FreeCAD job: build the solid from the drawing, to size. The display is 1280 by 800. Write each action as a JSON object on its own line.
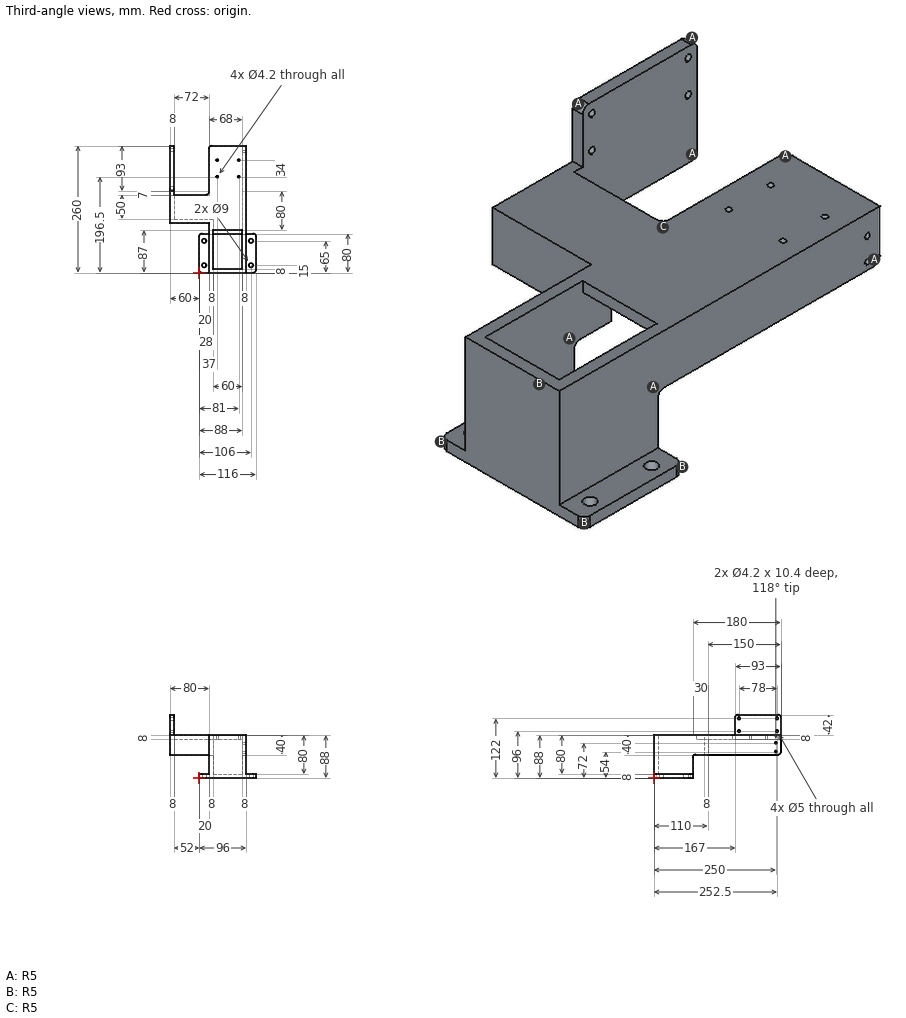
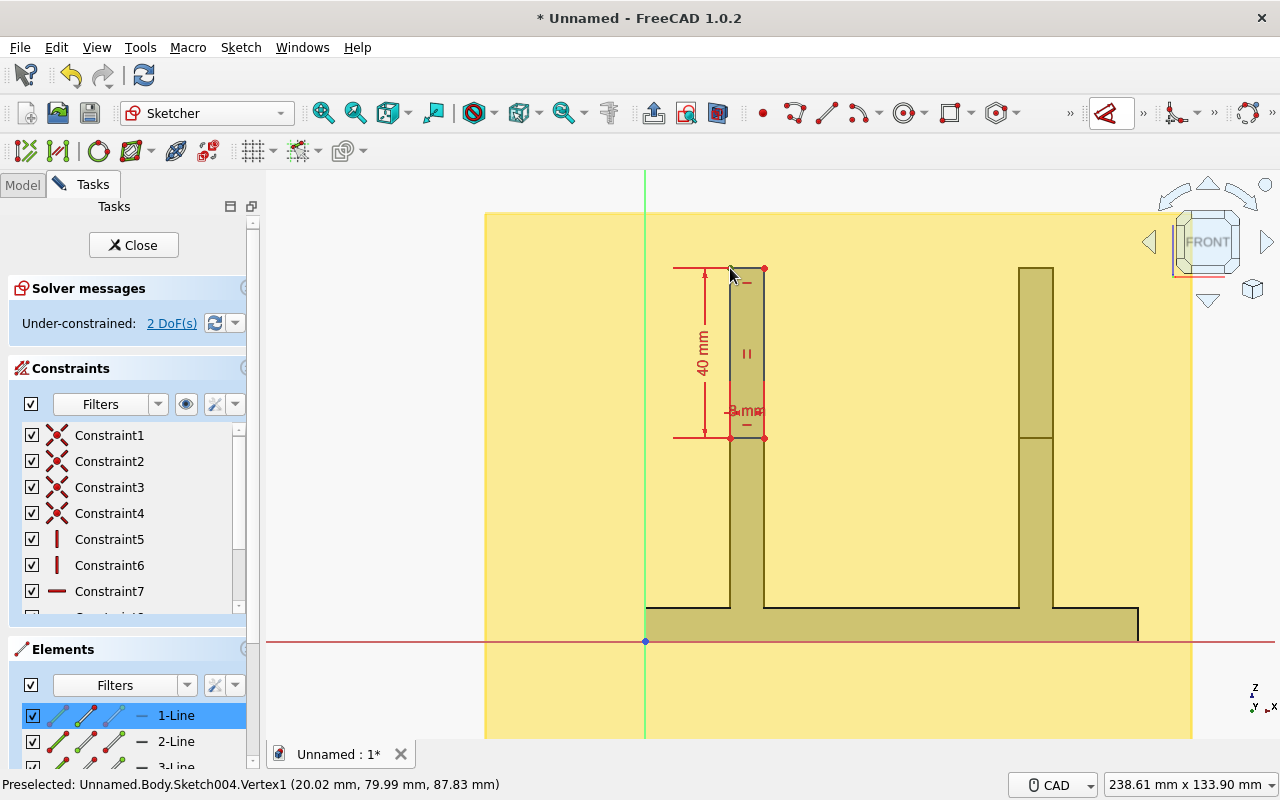
{"action": "left_click", "coordinate": [1128, 114]}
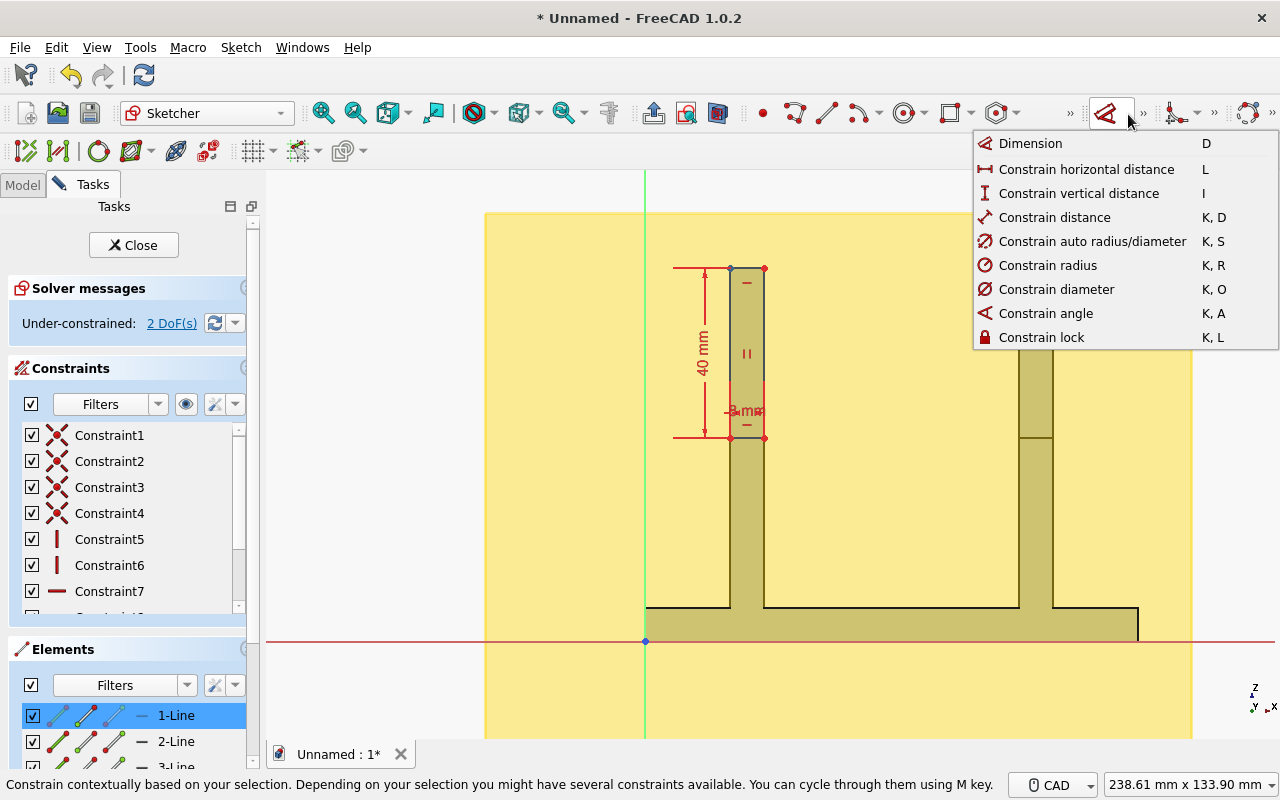
{"action": "left_click", "coordinate": [1126, 169]}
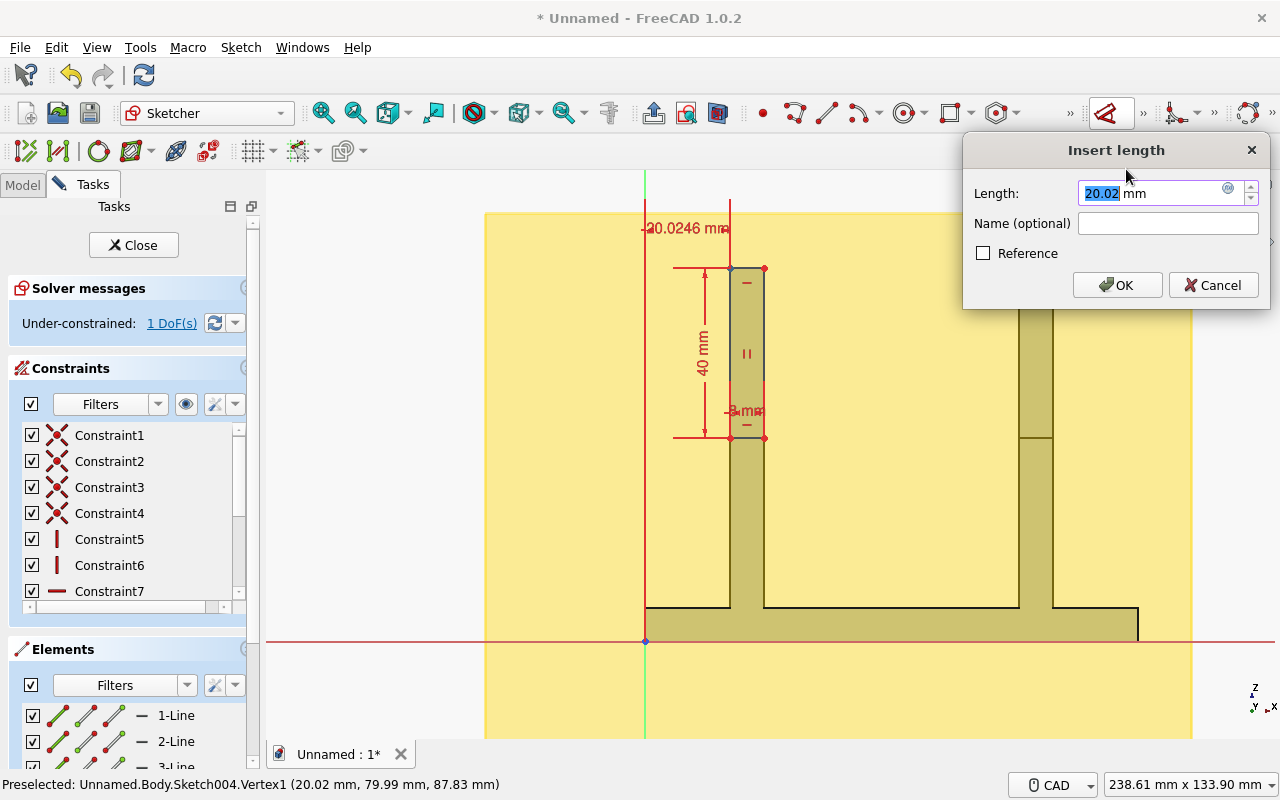
{"action": "type", "text": "20"}
{"action": "key", "text": "Return"}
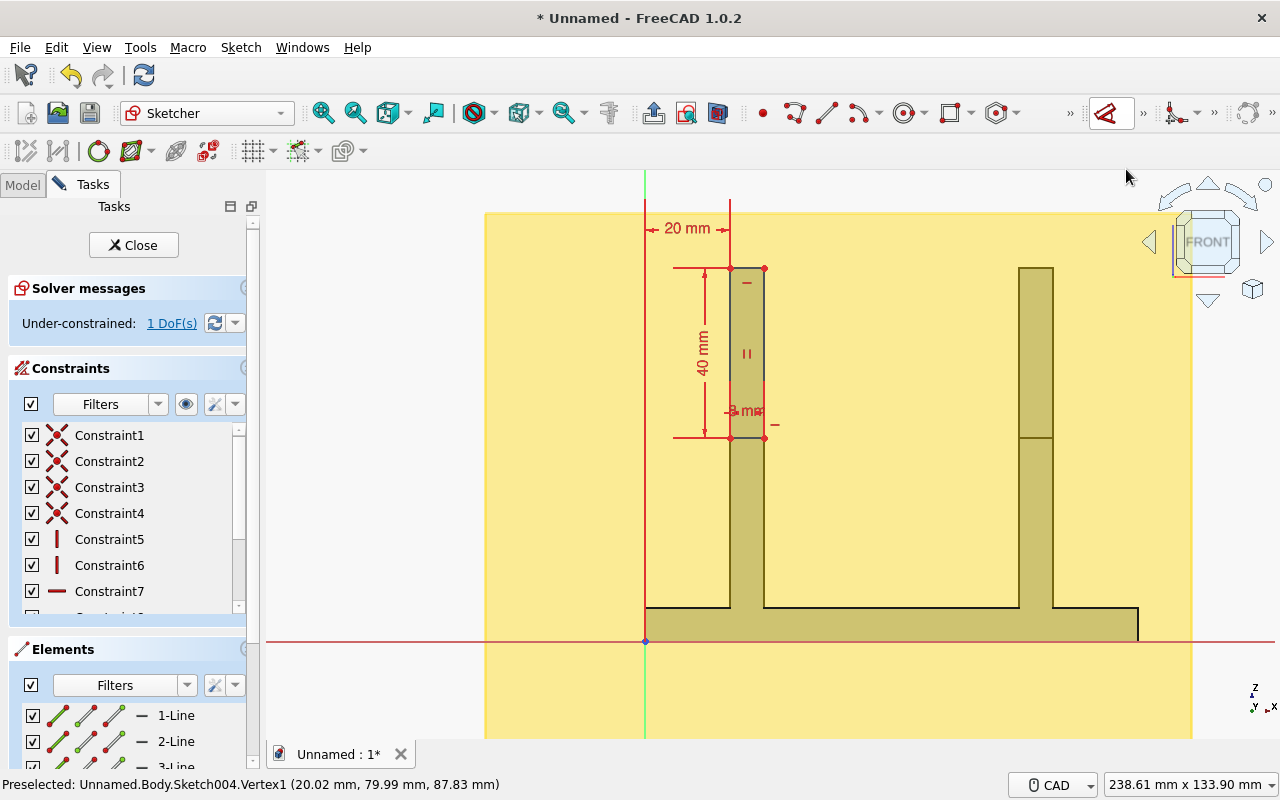
{"action": "left_click", "coordinate": [730, 268]}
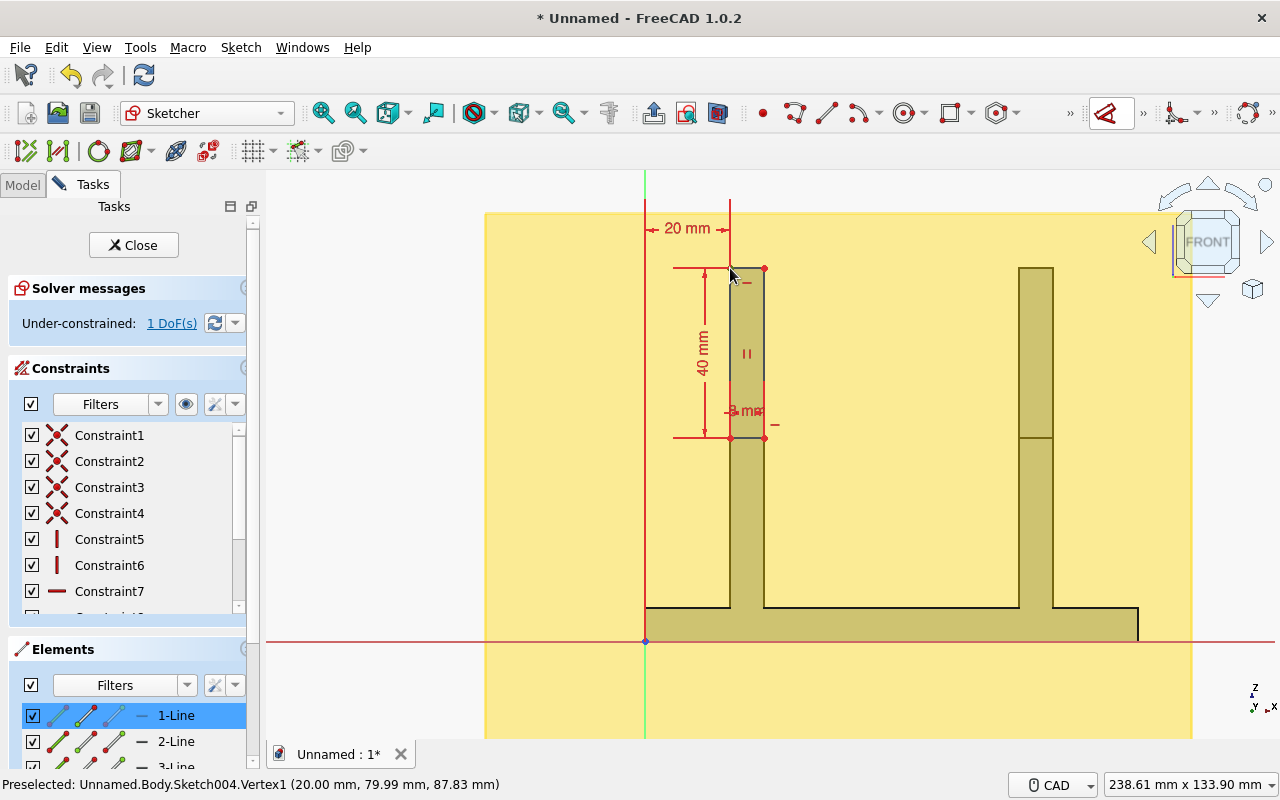
{"action": "key", "text": "i"}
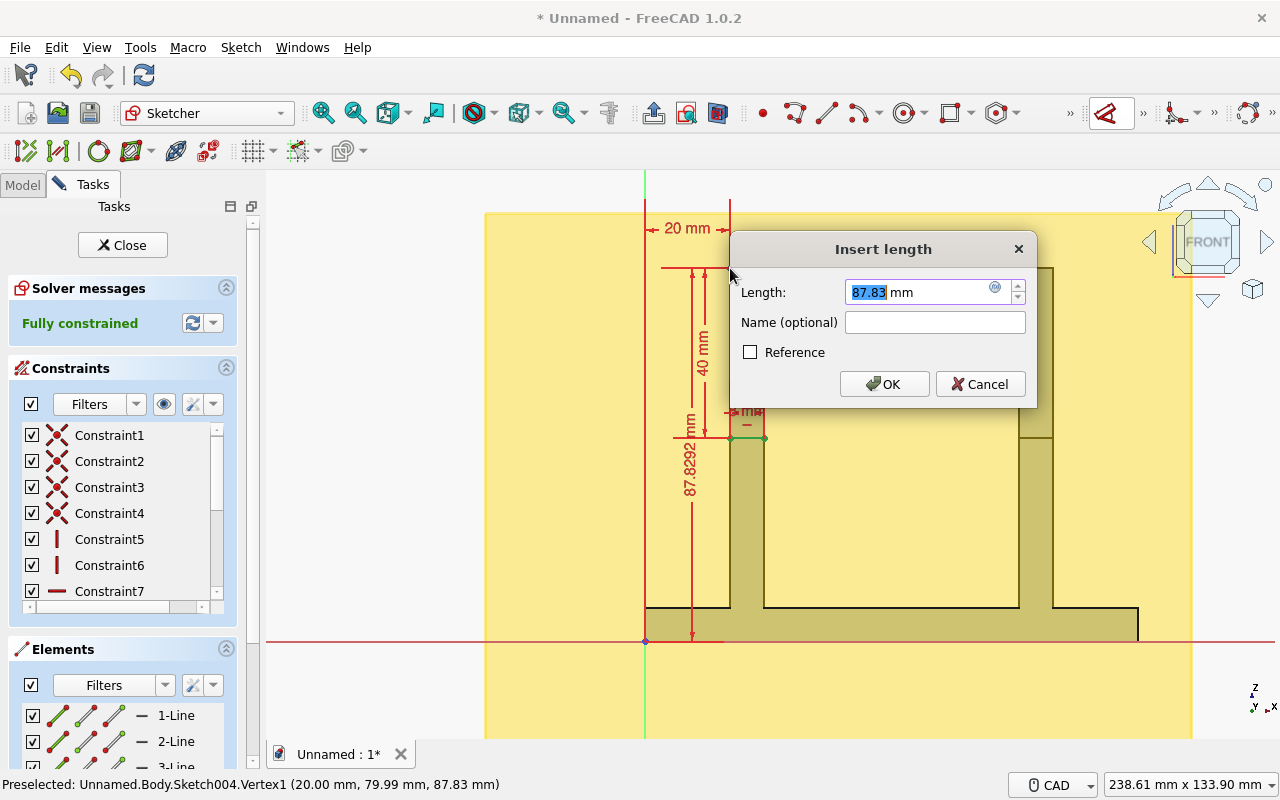
{"action": "type", "text": "88"}
{"action": "key", "text": "Return"}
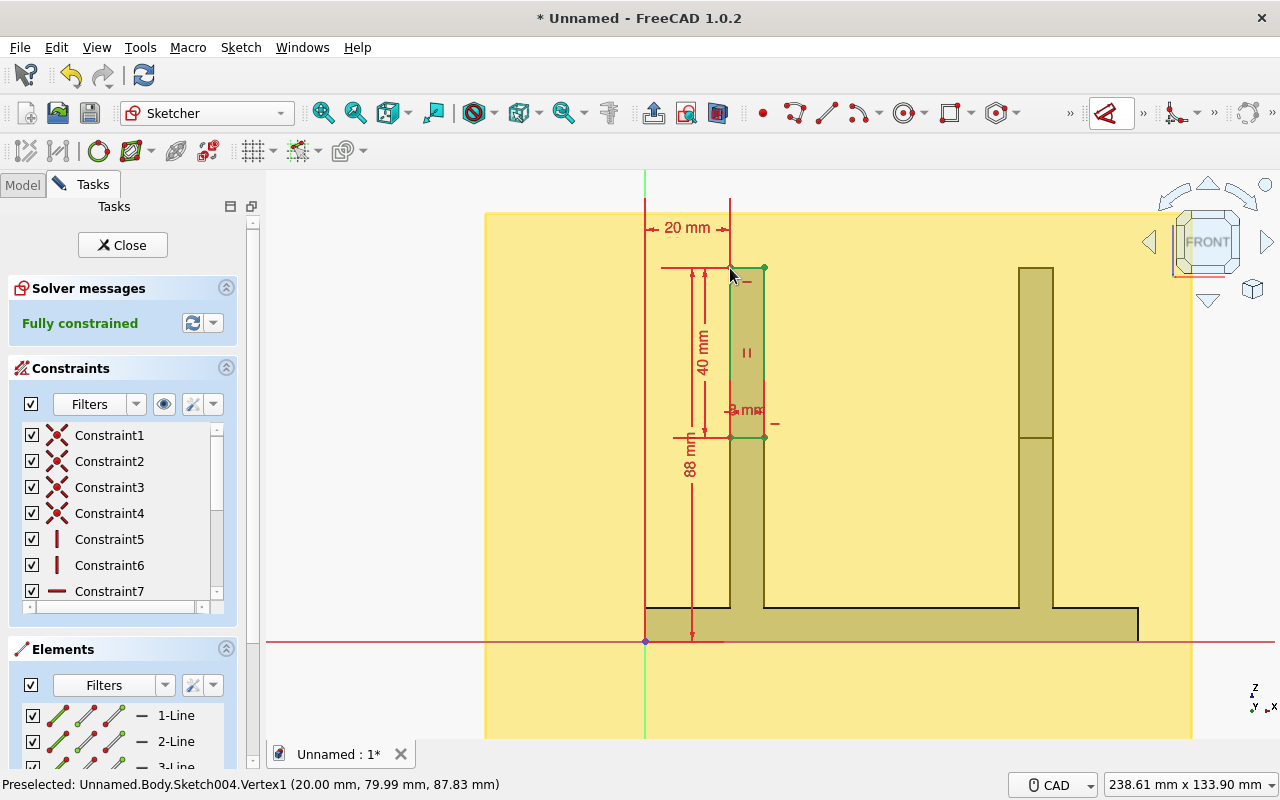
{"action": "left_click", "coordinate": [123, 245]}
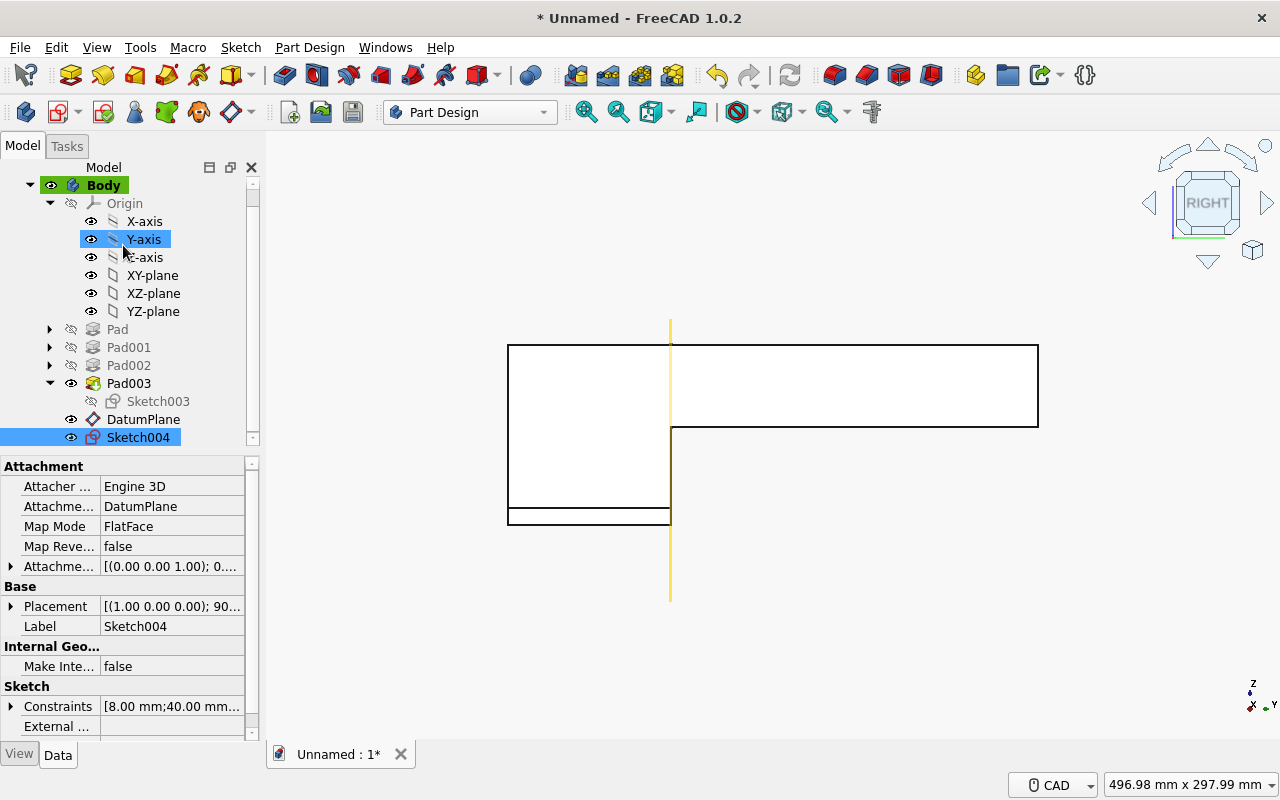
{"action": "left_click", "coordinate": [72, 76]}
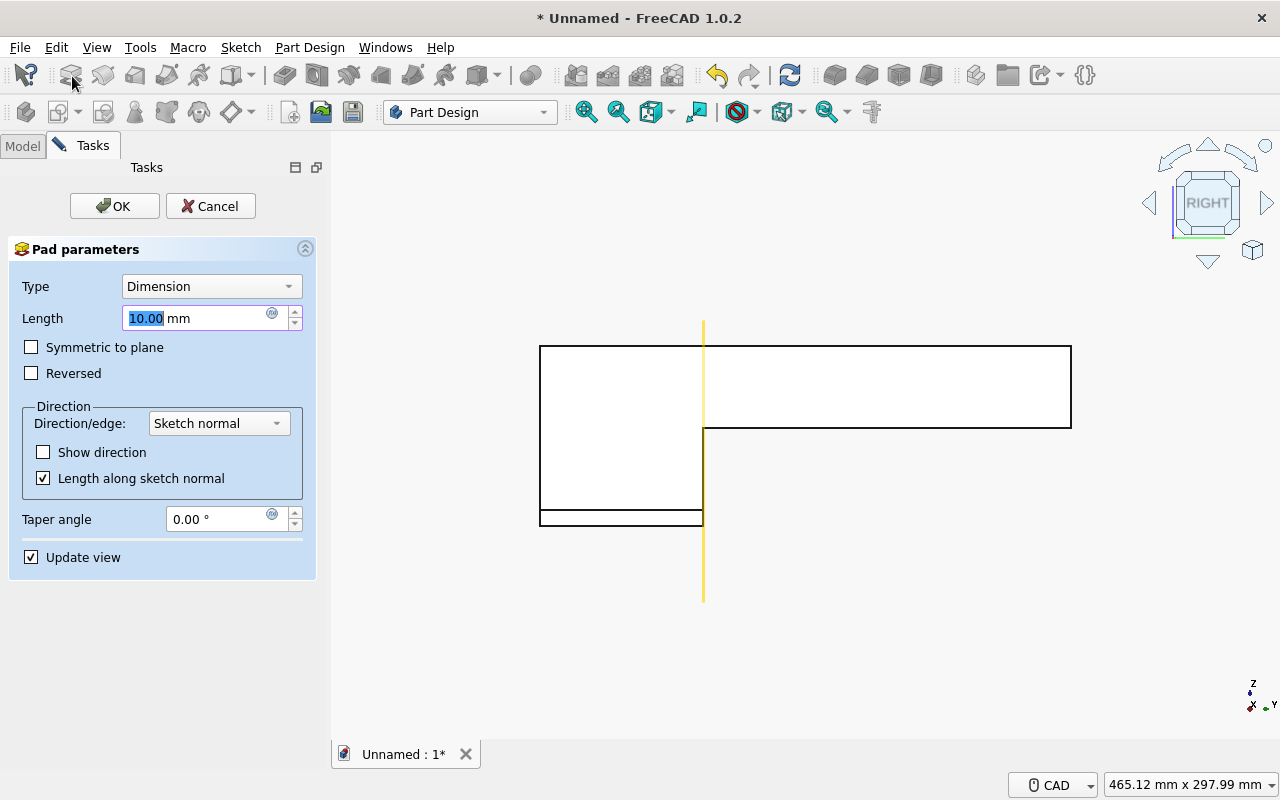
{"action": "type", "text": "30"}
{"action": "key", "text": "Tab"}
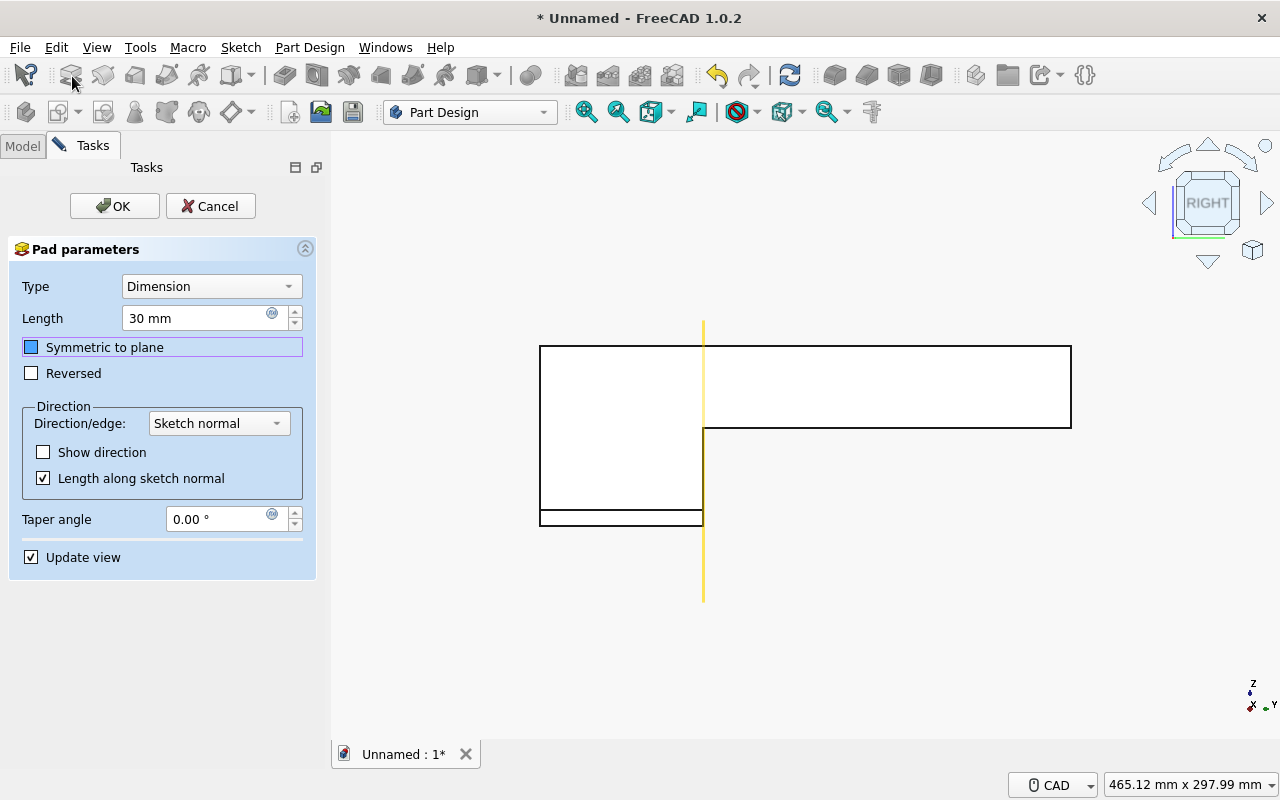
{"action": "left_click", "coordinate": [30, 373]}